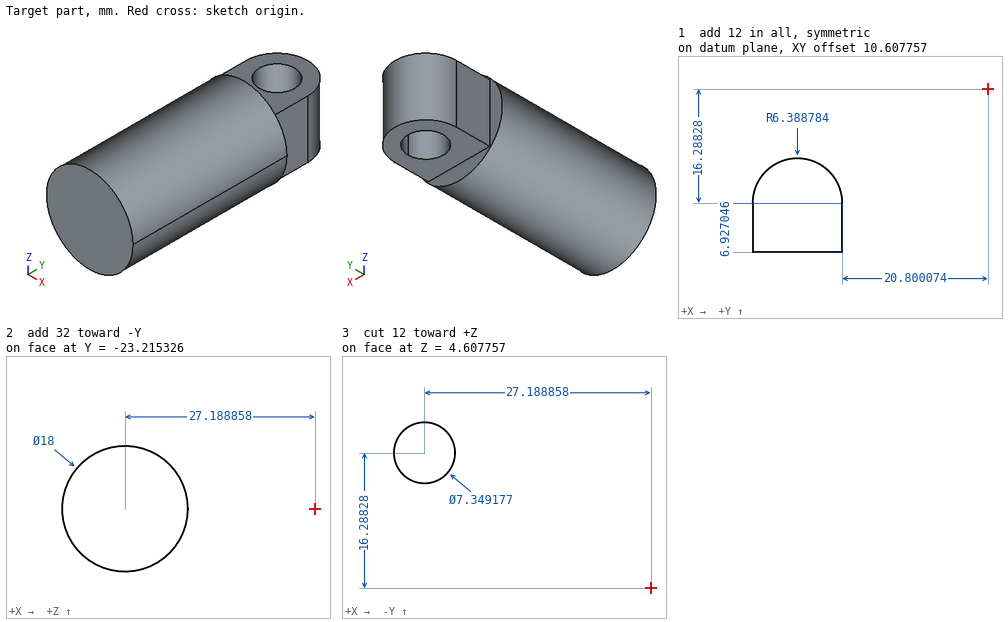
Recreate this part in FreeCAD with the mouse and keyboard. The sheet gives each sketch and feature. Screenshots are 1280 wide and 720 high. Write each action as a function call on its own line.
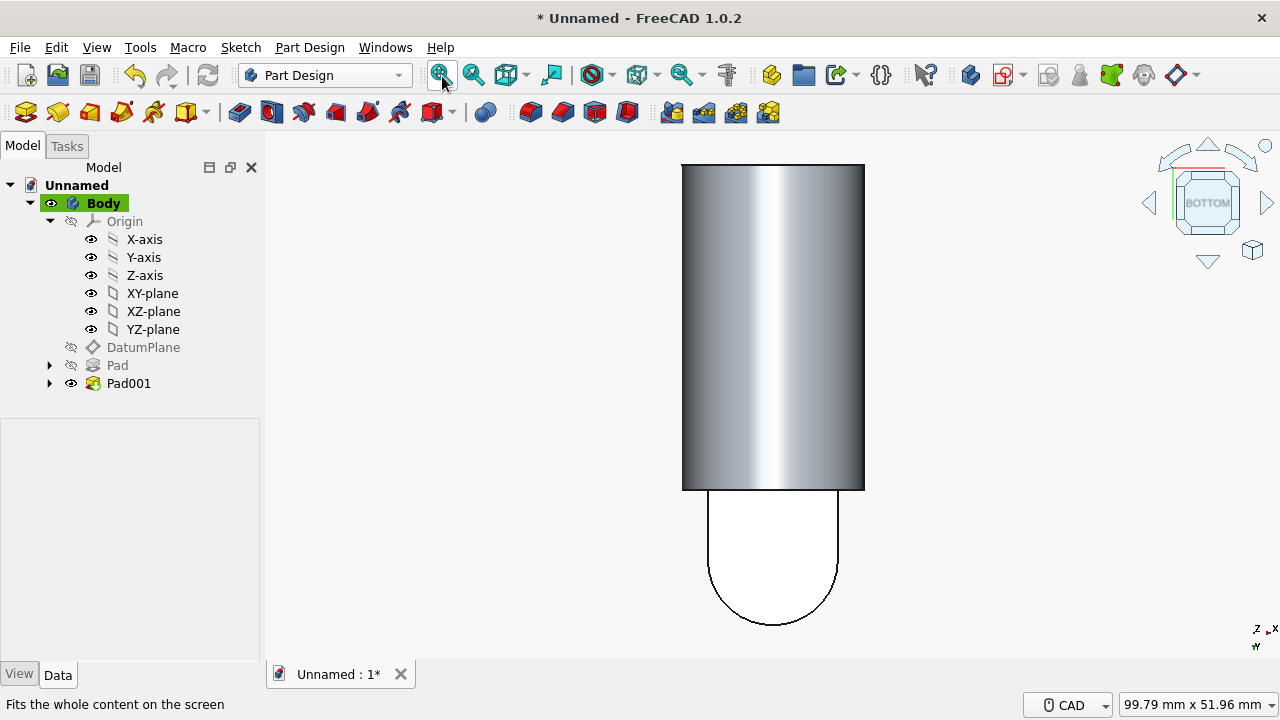
click(773, 557)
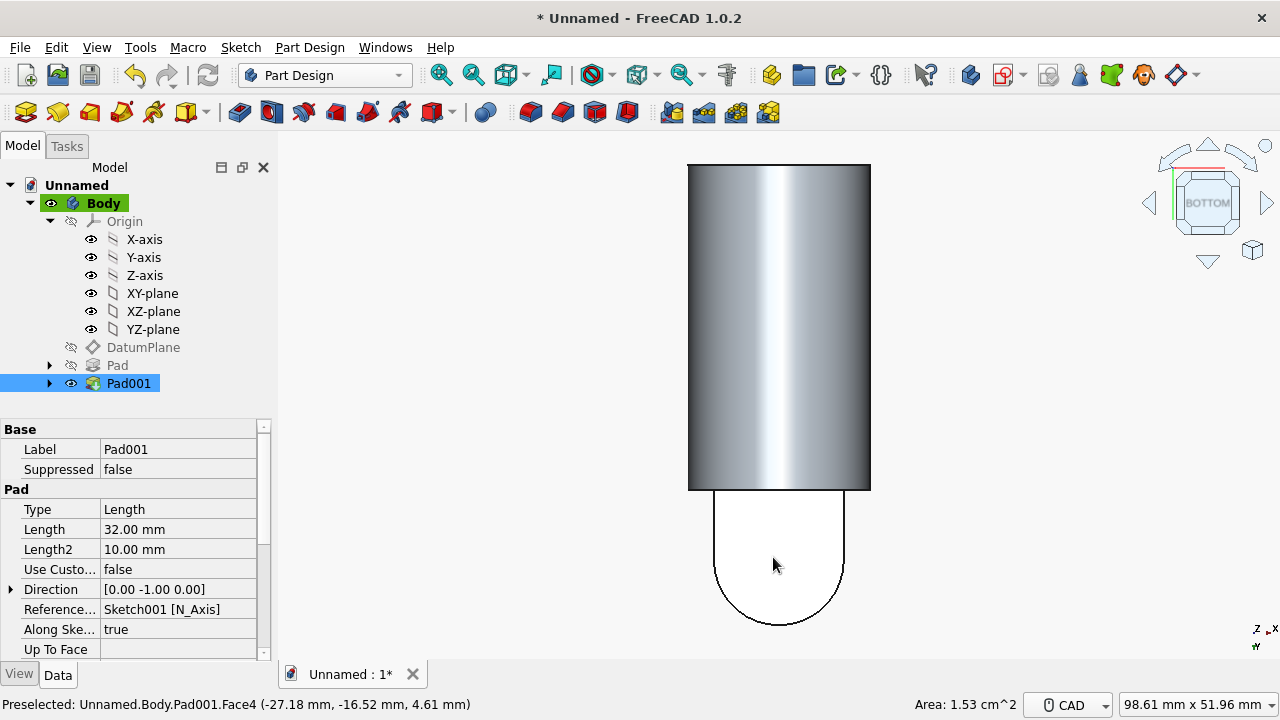
click(1004, 76)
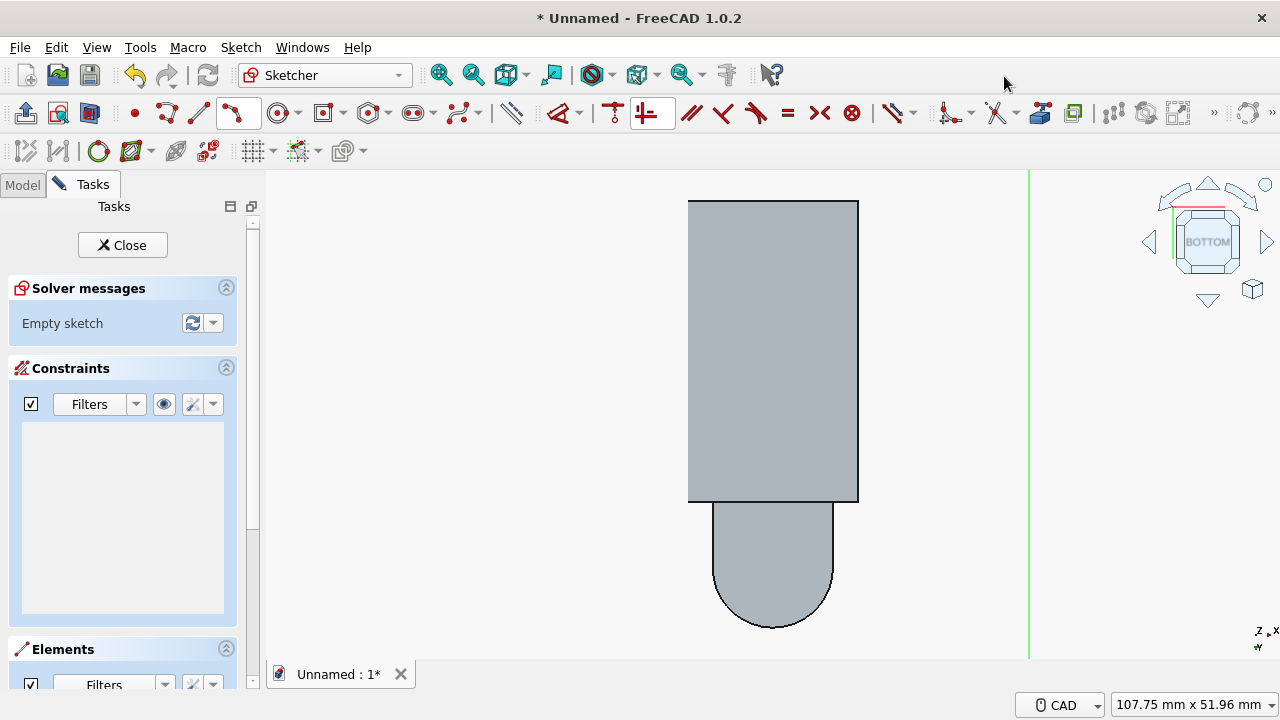
scroll(795, 618, up, 7)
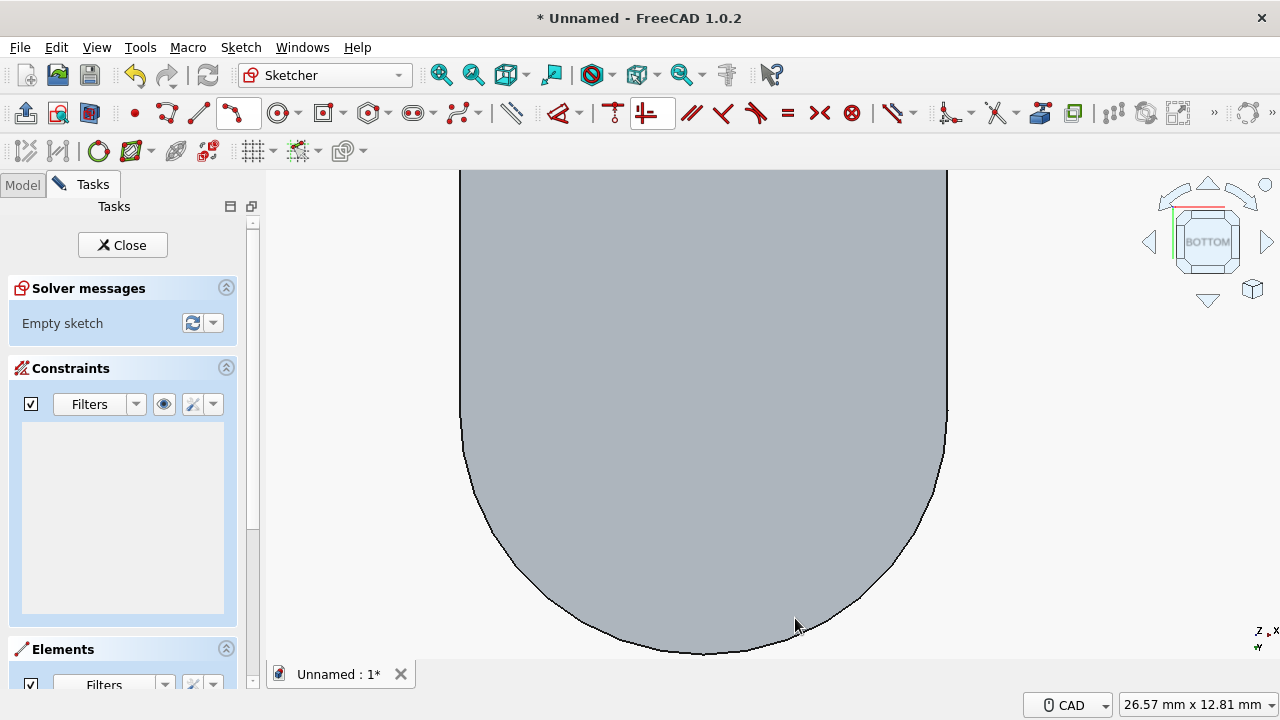
click(278, 114)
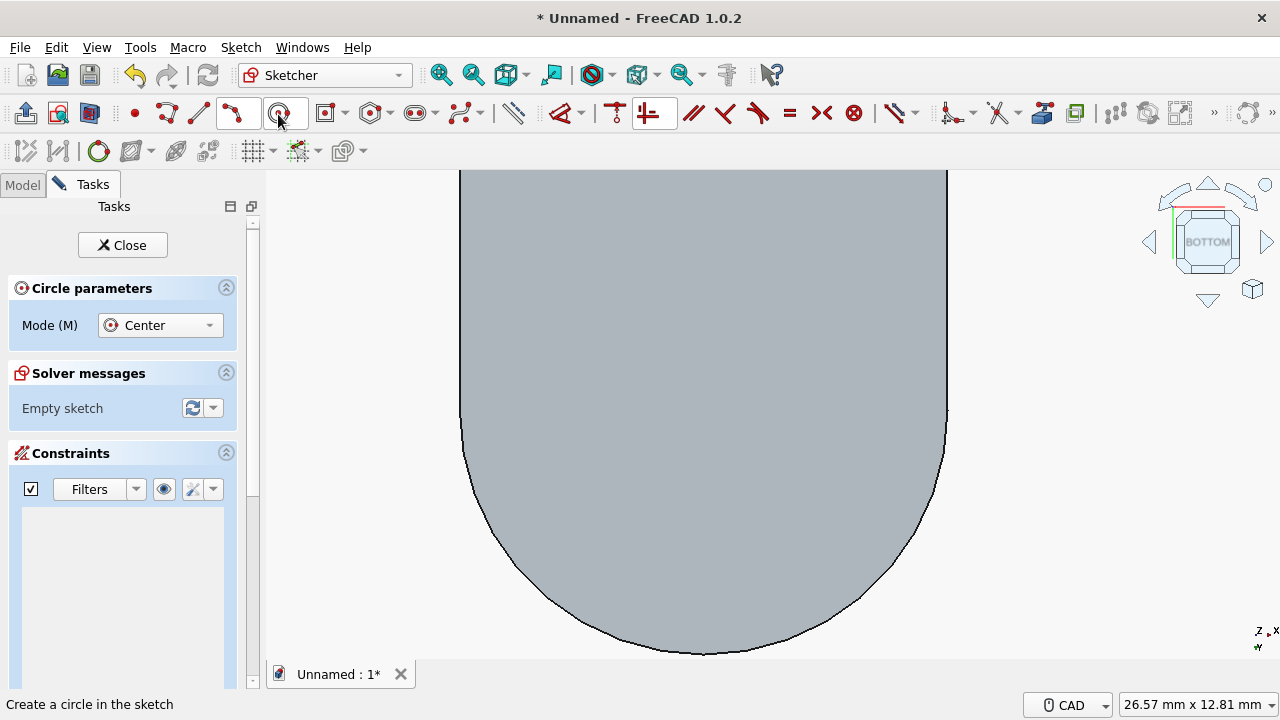
click(704, 411)
move(803, 312)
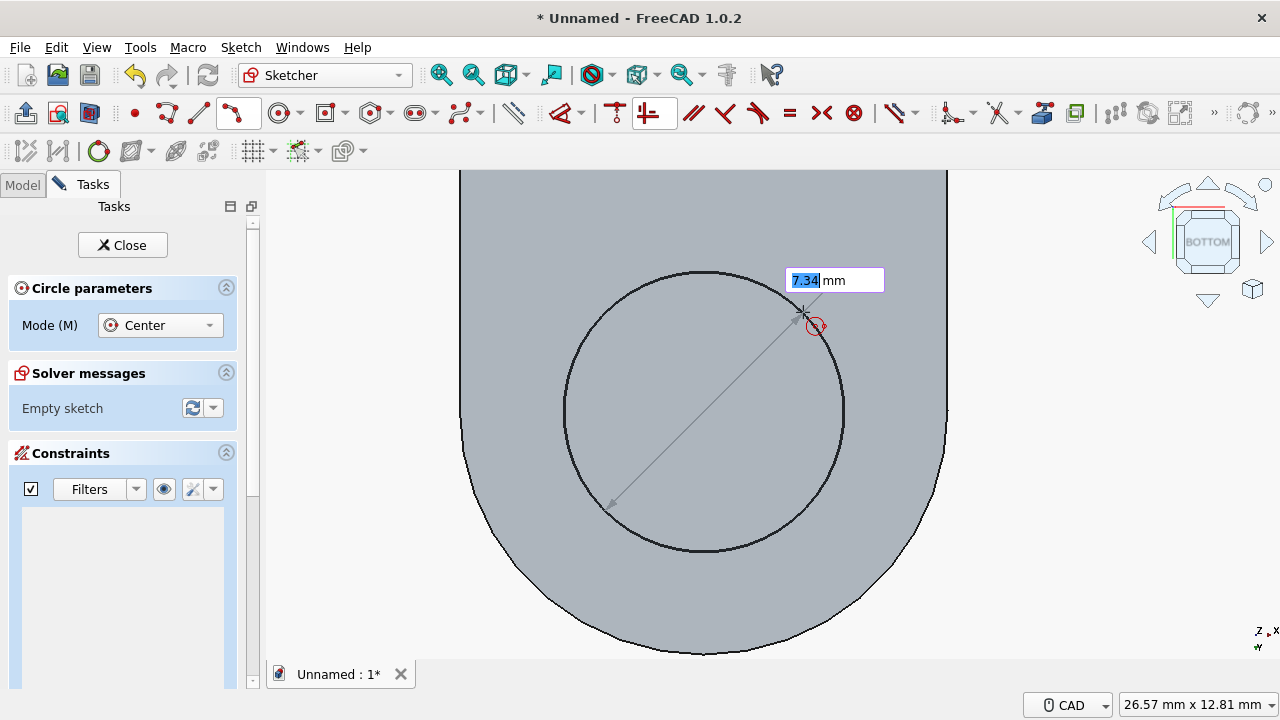
text(7.349177)
key(Return)
key(Escape)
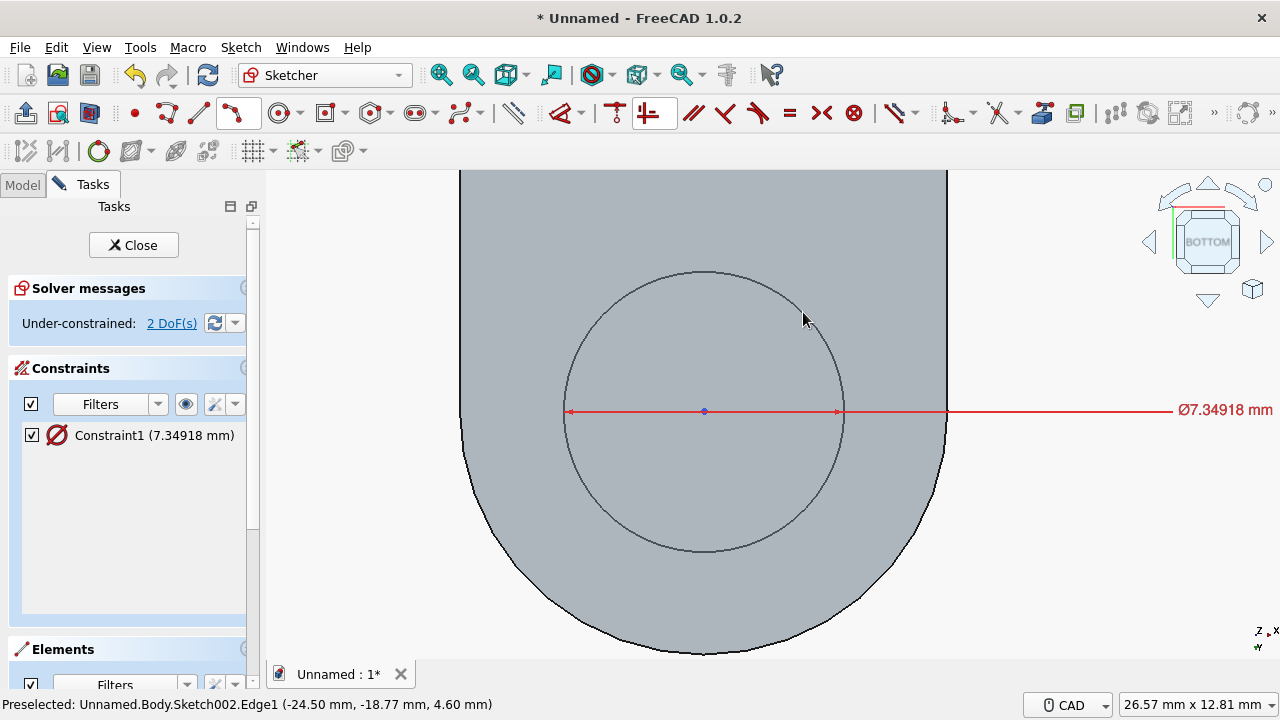
click(560, 114)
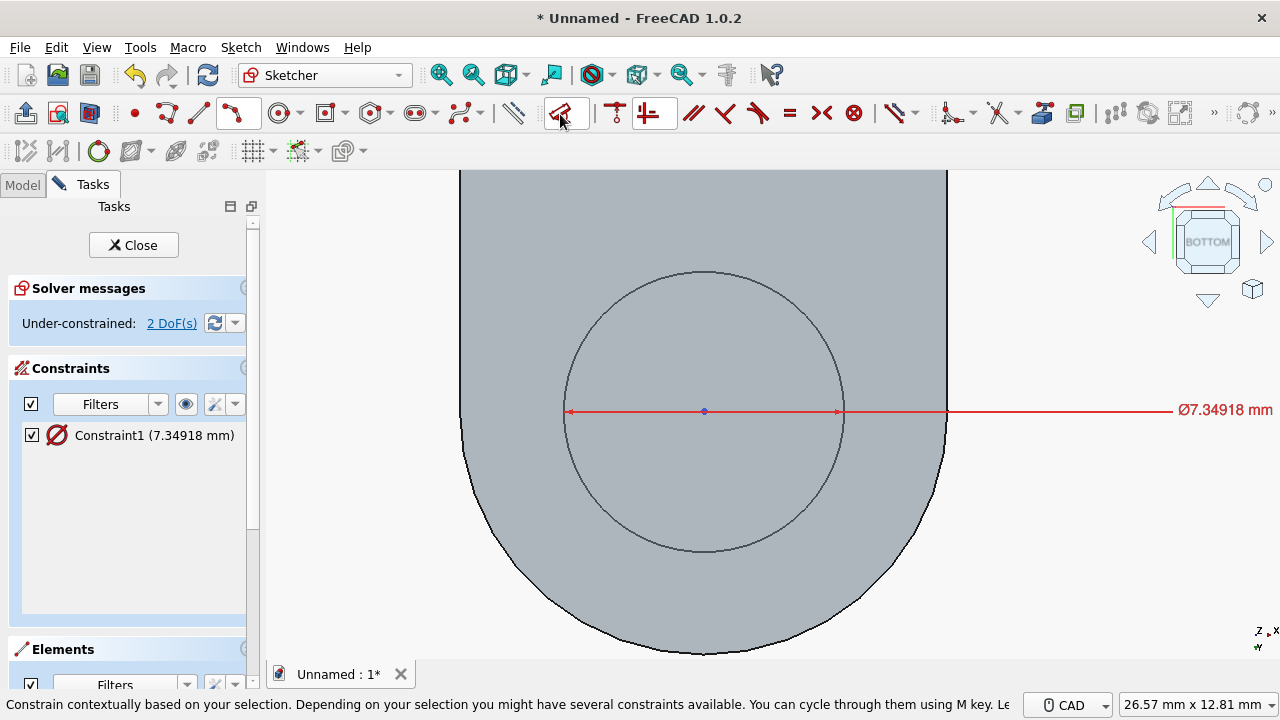
click(704, 412)
click(670, 522)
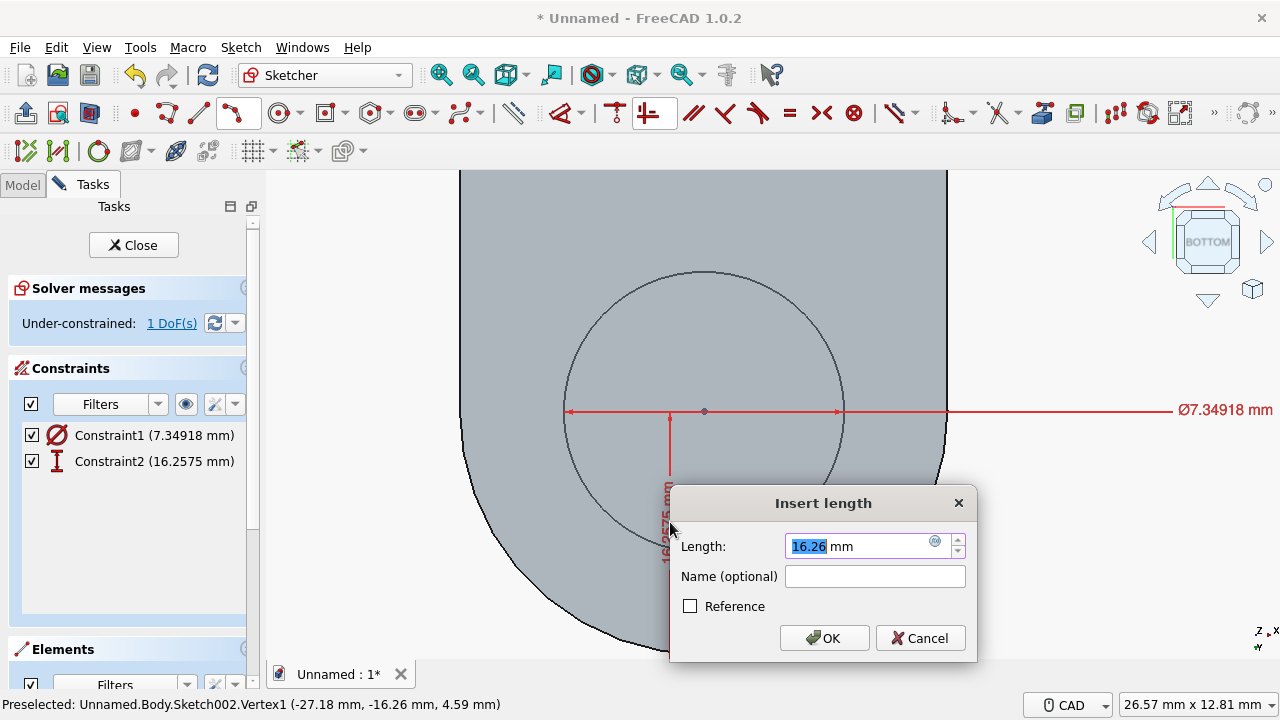
text(16.28828)
key(Return)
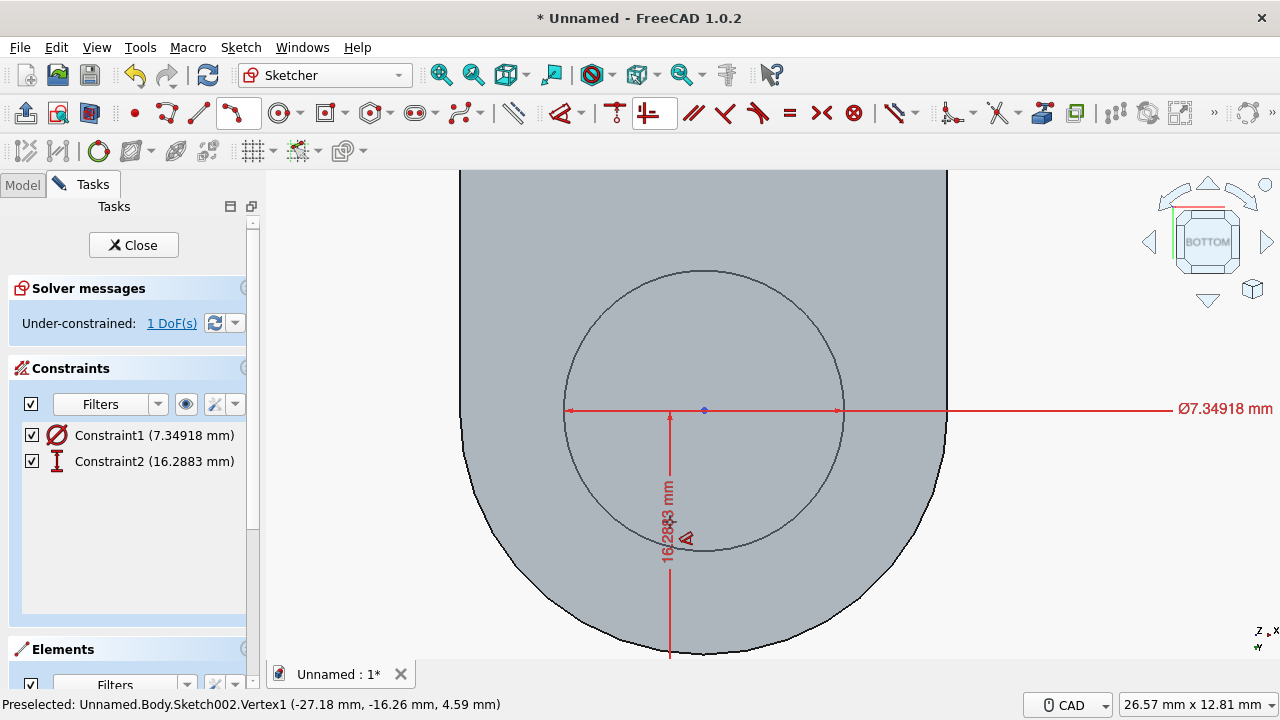
click(704, 411)
click(909, 377)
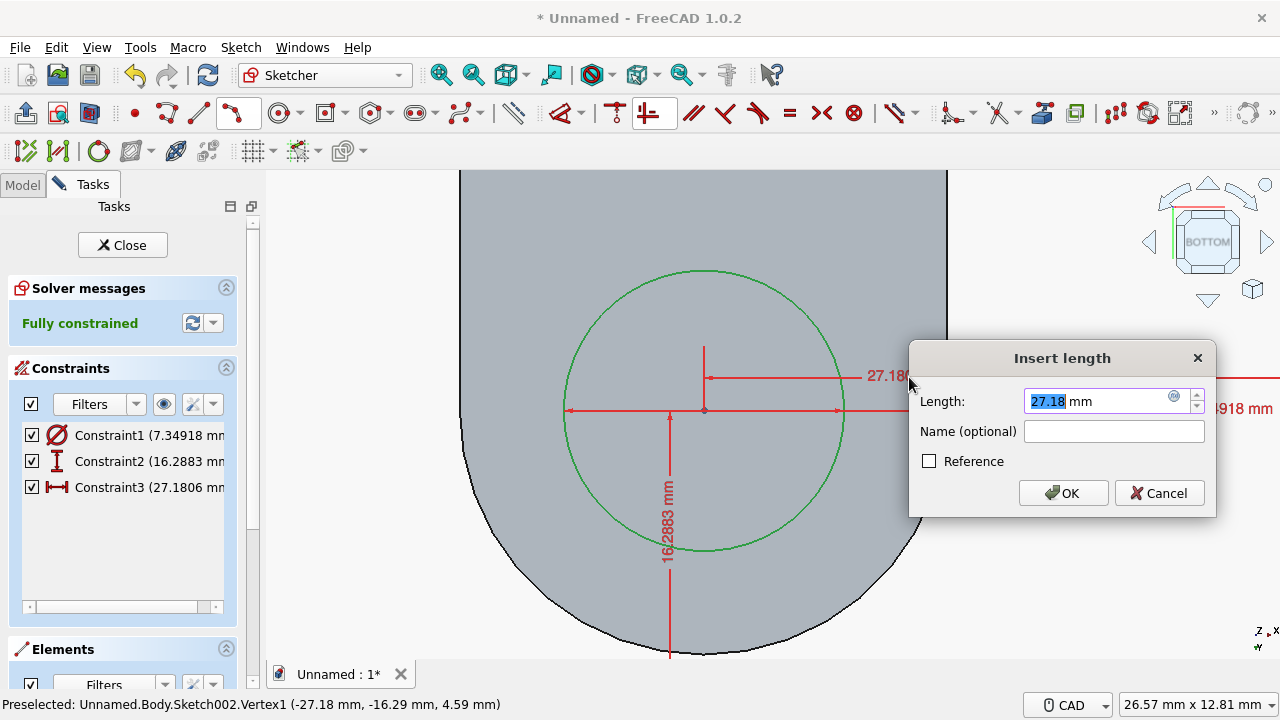
text(27.188858)
key(Return)
key(Escape)